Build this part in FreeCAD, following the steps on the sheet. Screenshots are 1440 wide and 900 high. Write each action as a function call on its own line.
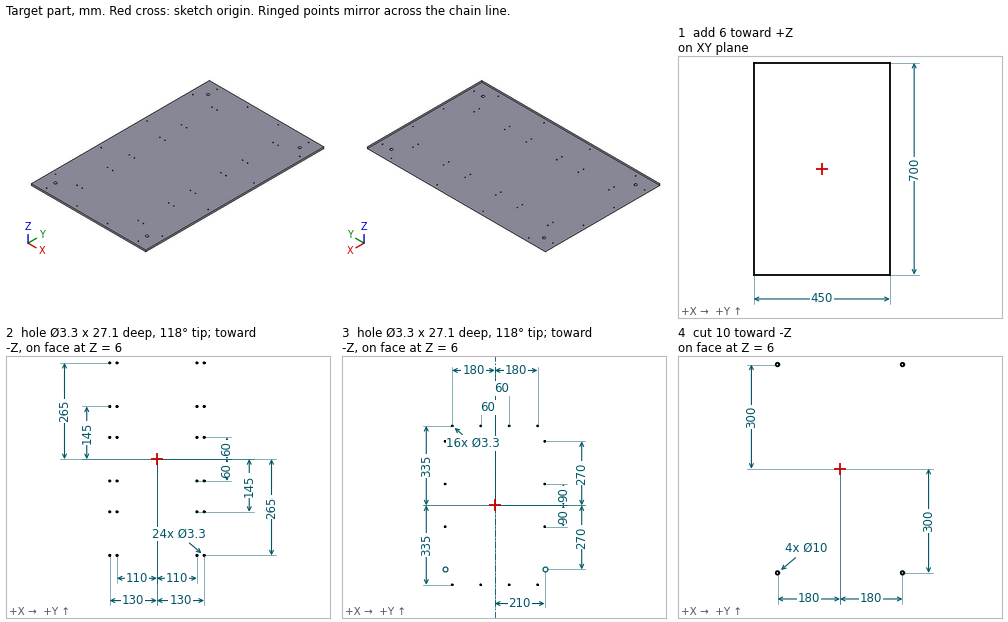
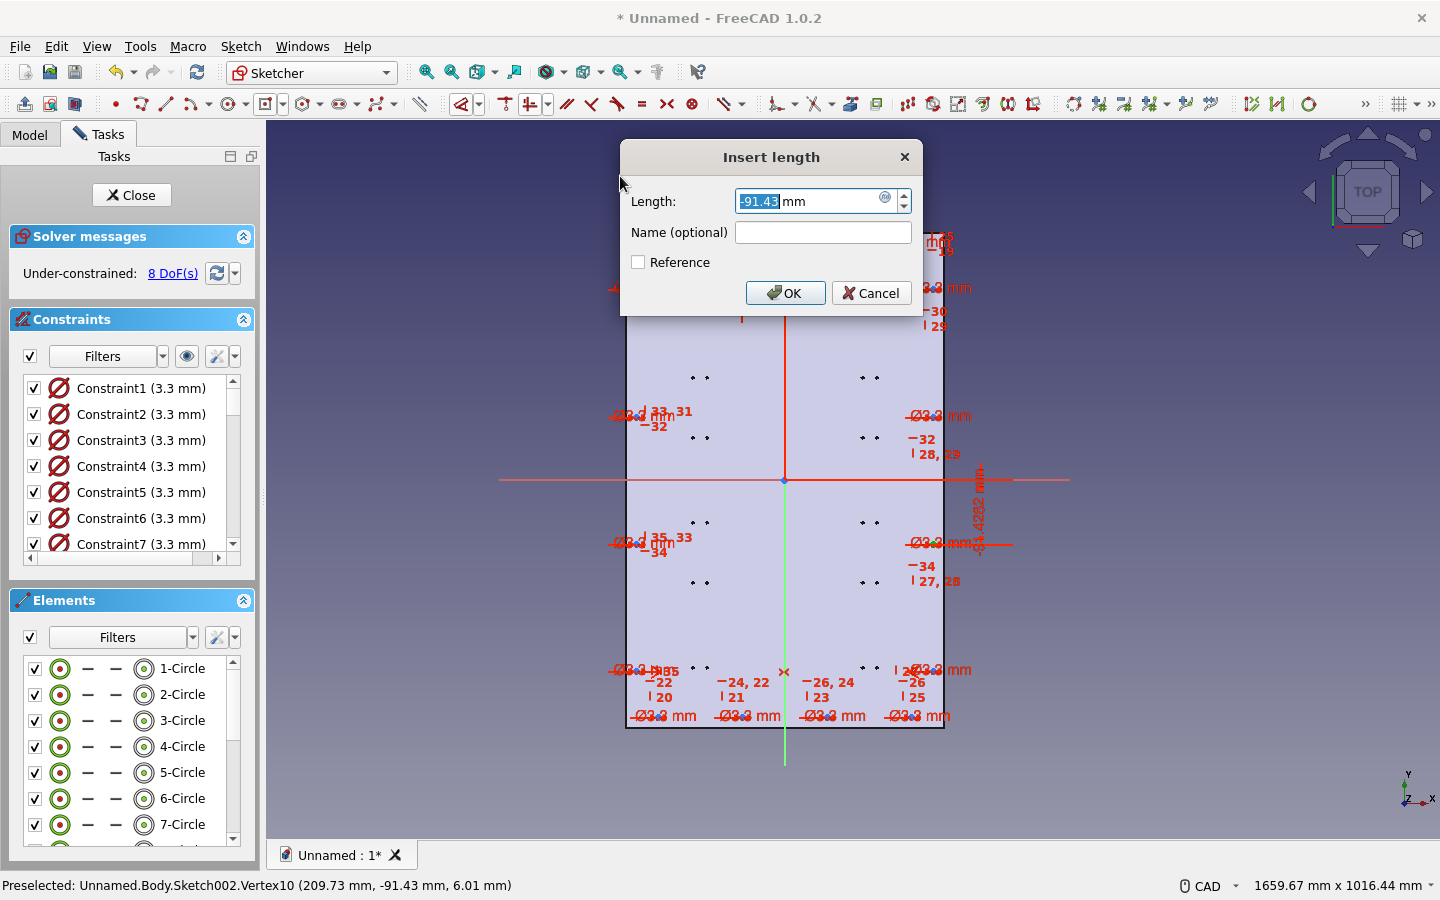
text(-90)
key(Return)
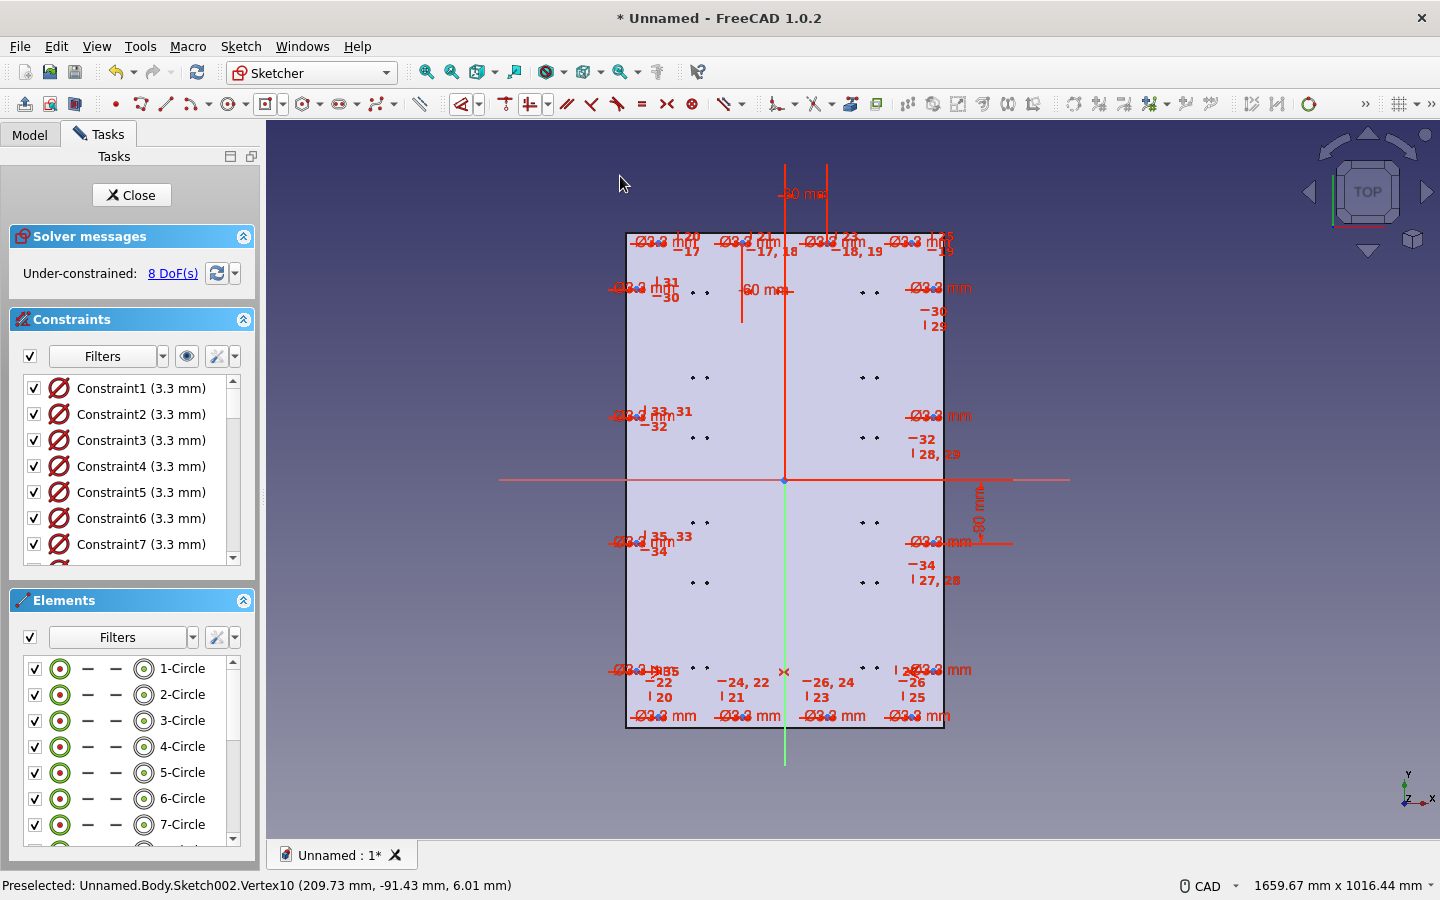
click(933, 418)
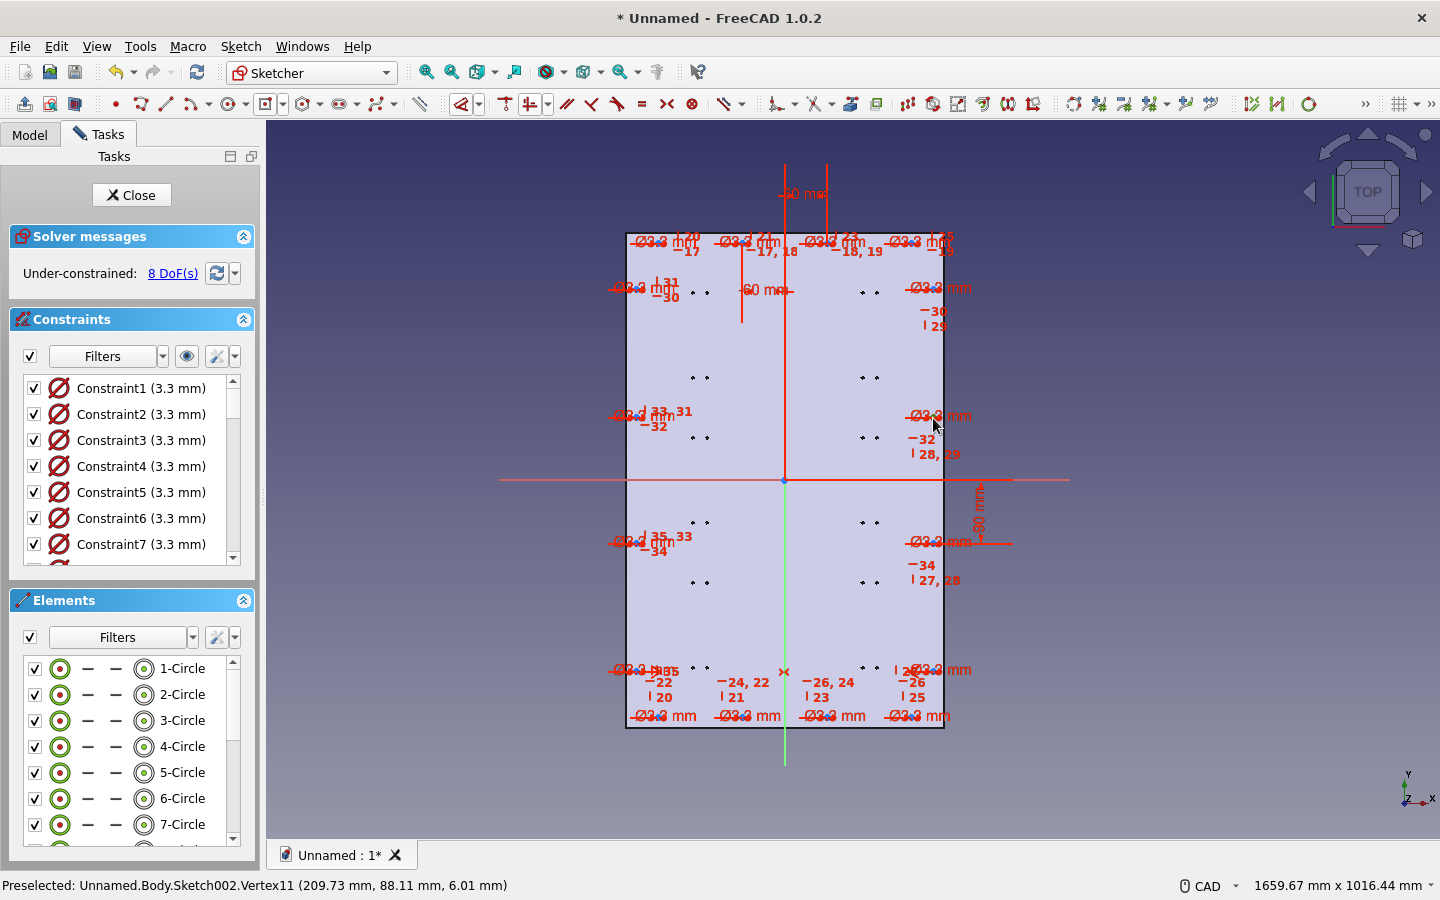
key(i)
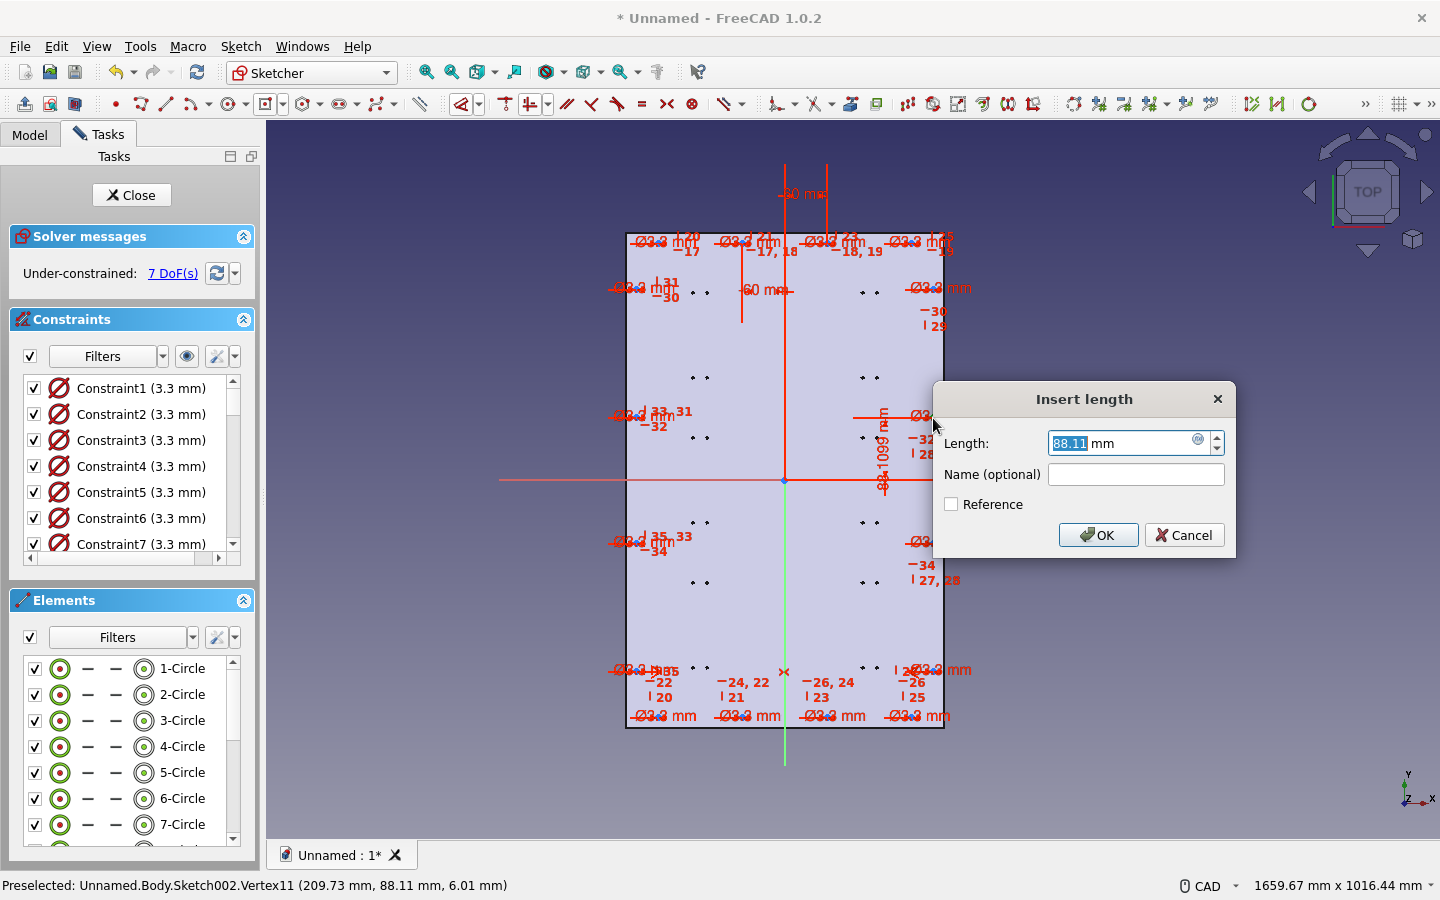
text(90)
key(Return)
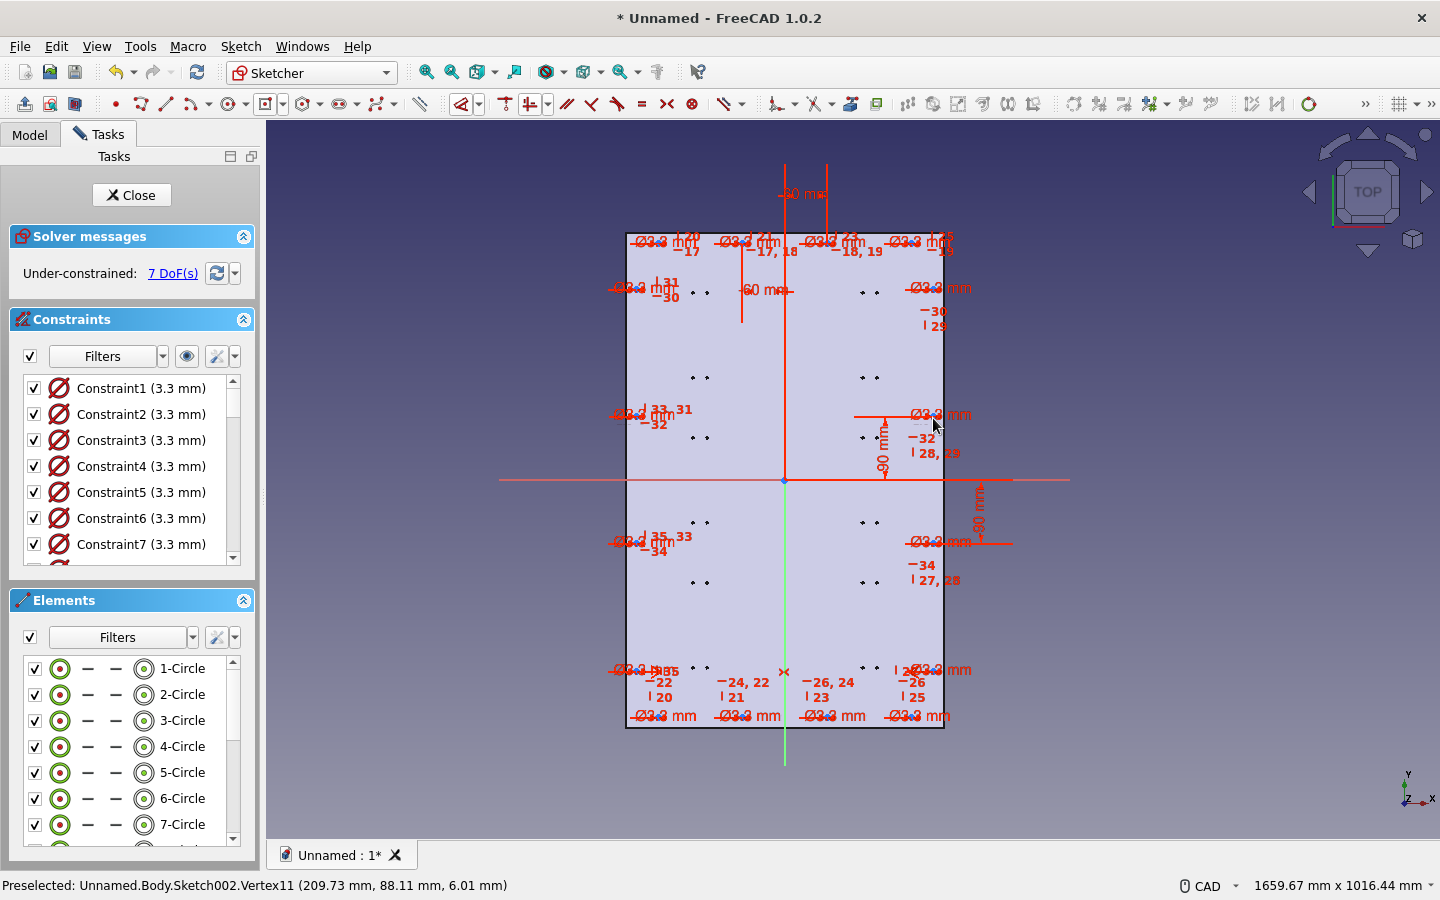
click(658, 244)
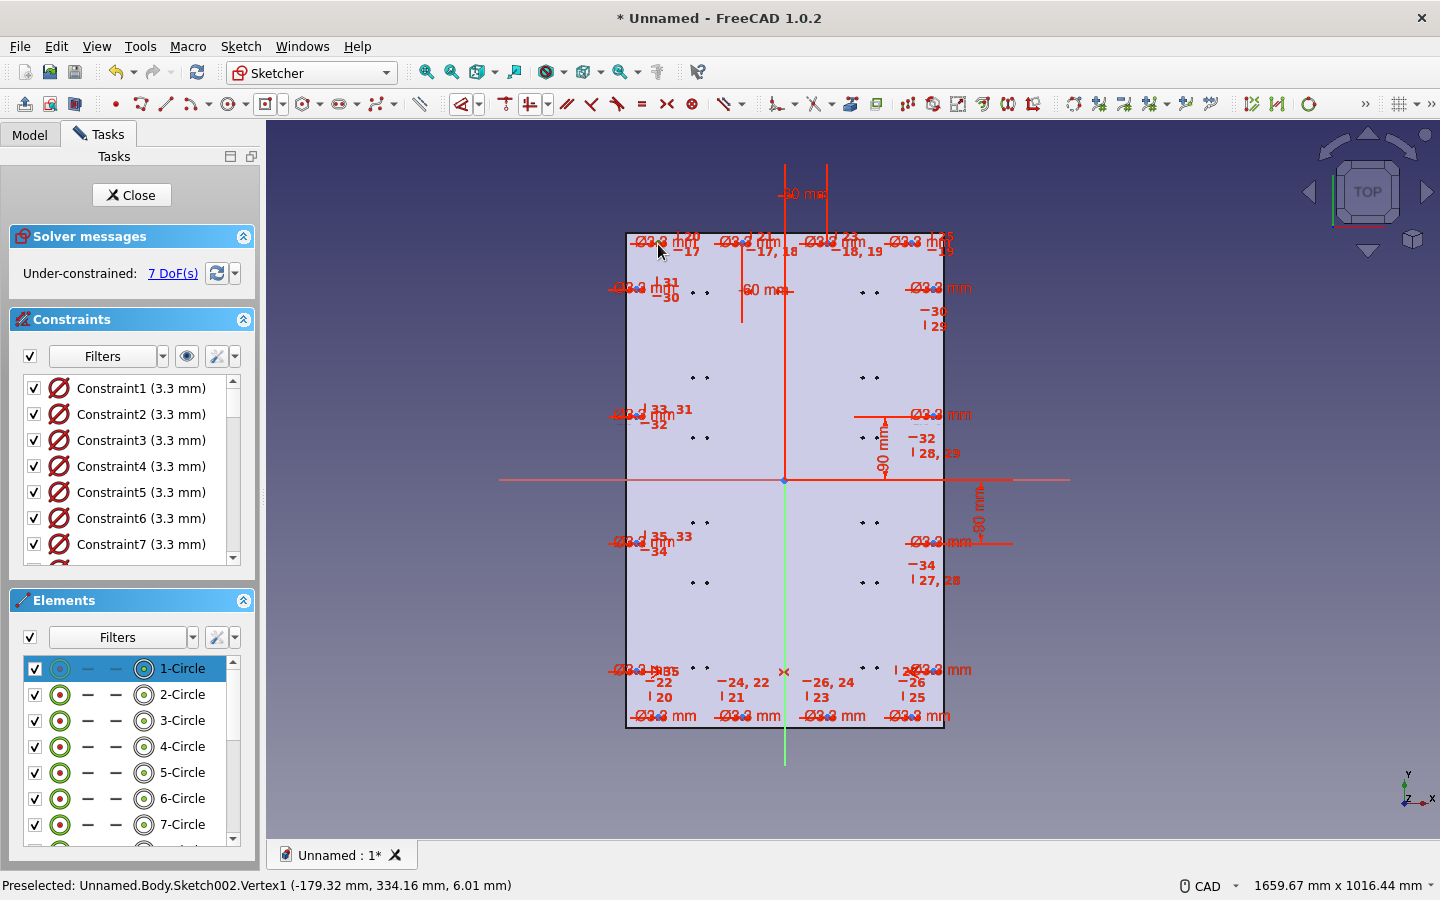
key(l)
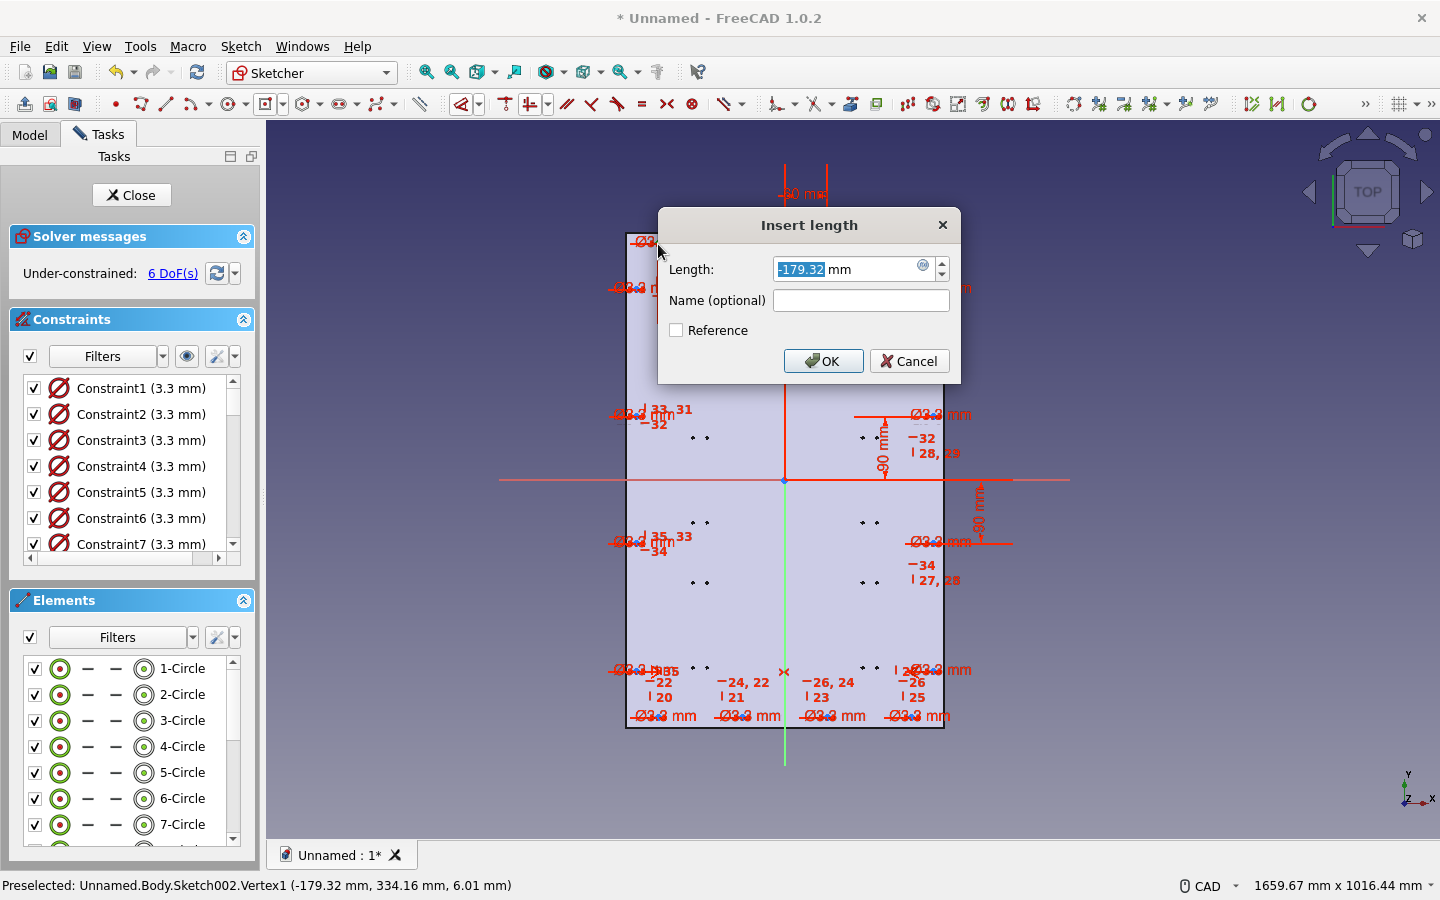
text(-180)
key(Return)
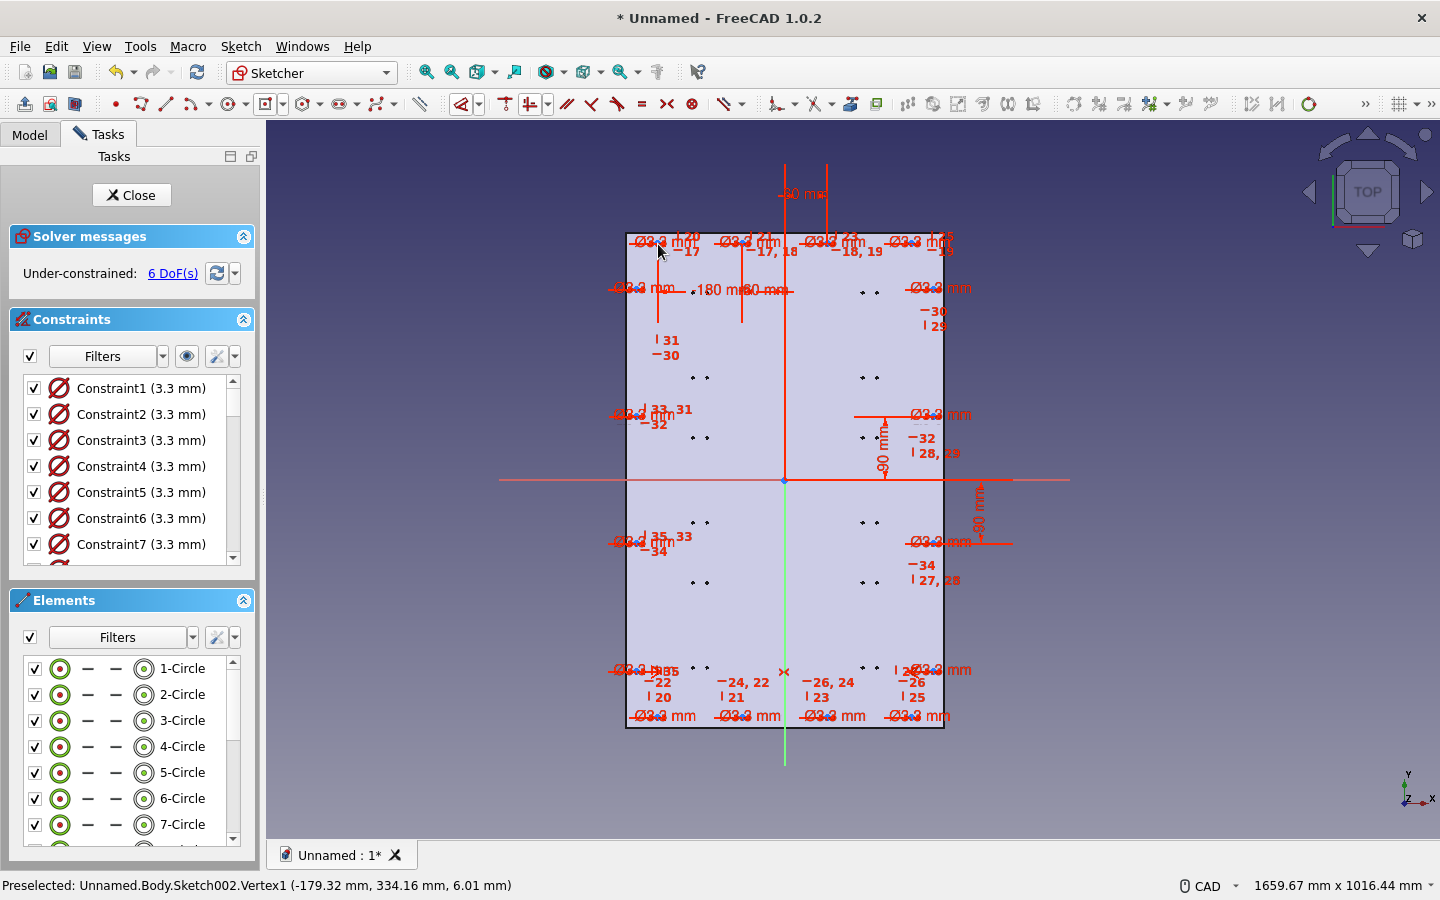
click(658, 244)